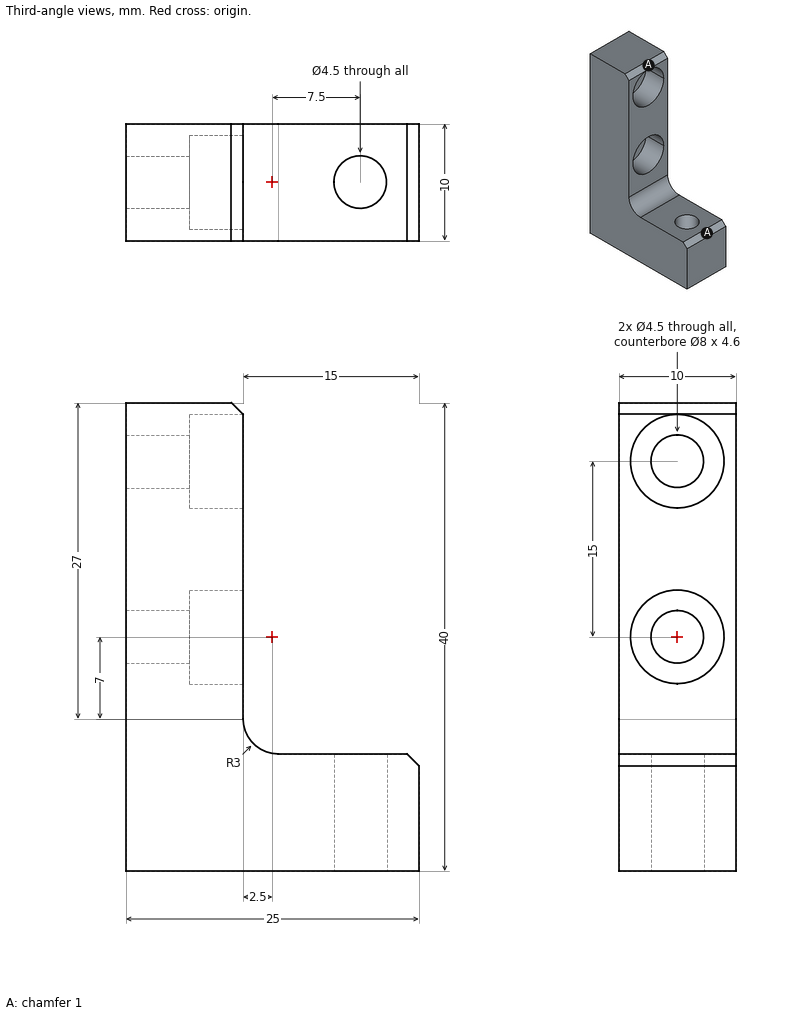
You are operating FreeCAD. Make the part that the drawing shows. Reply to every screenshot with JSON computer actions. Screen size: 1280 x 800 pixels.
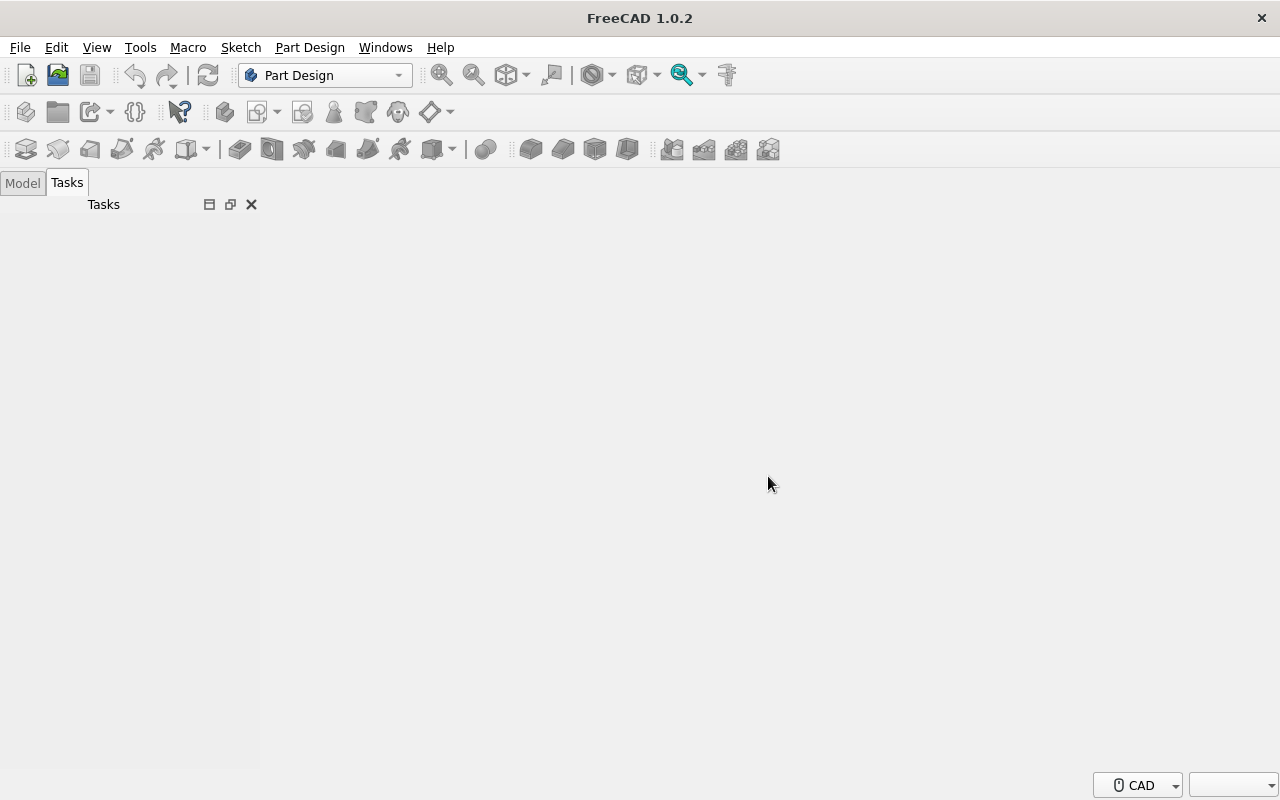
{"action": "left_click", "coordinate": [26, 76]}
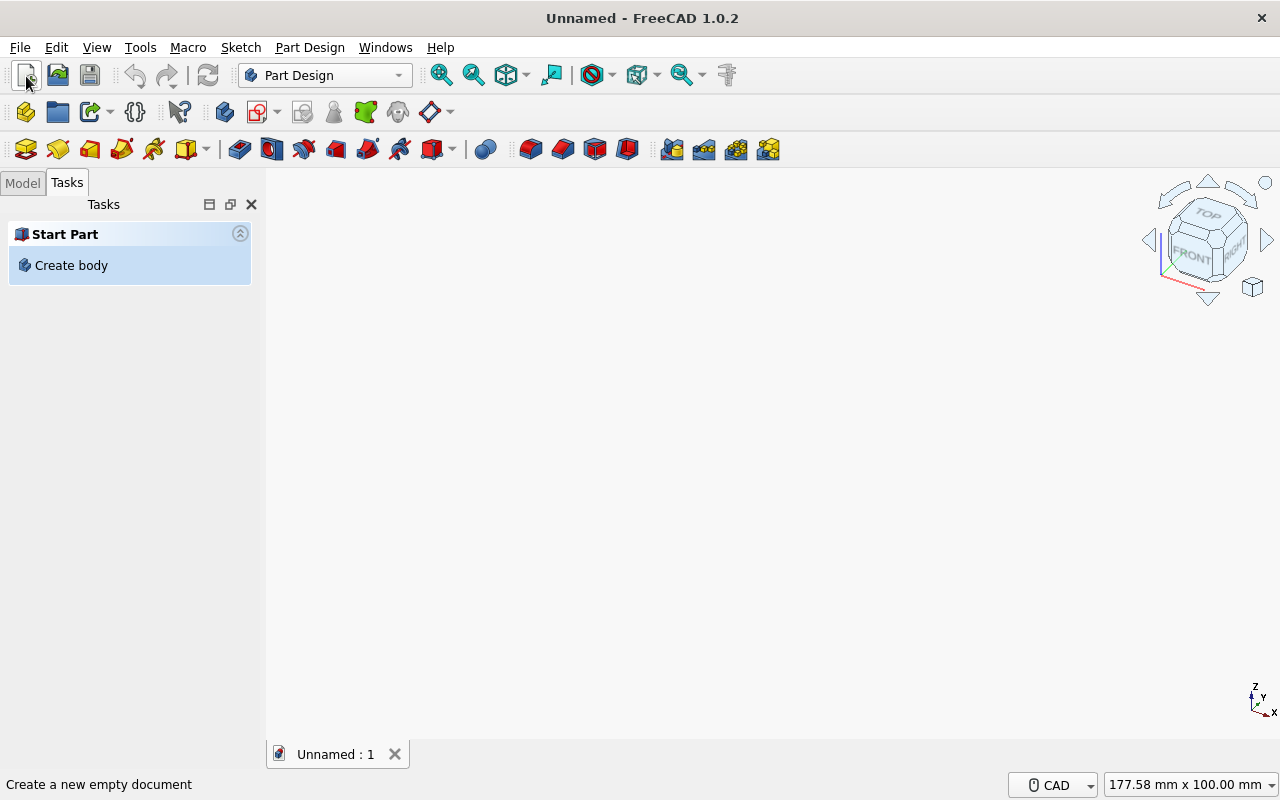
{"action": "left_click", "coordinate": [258, 112]}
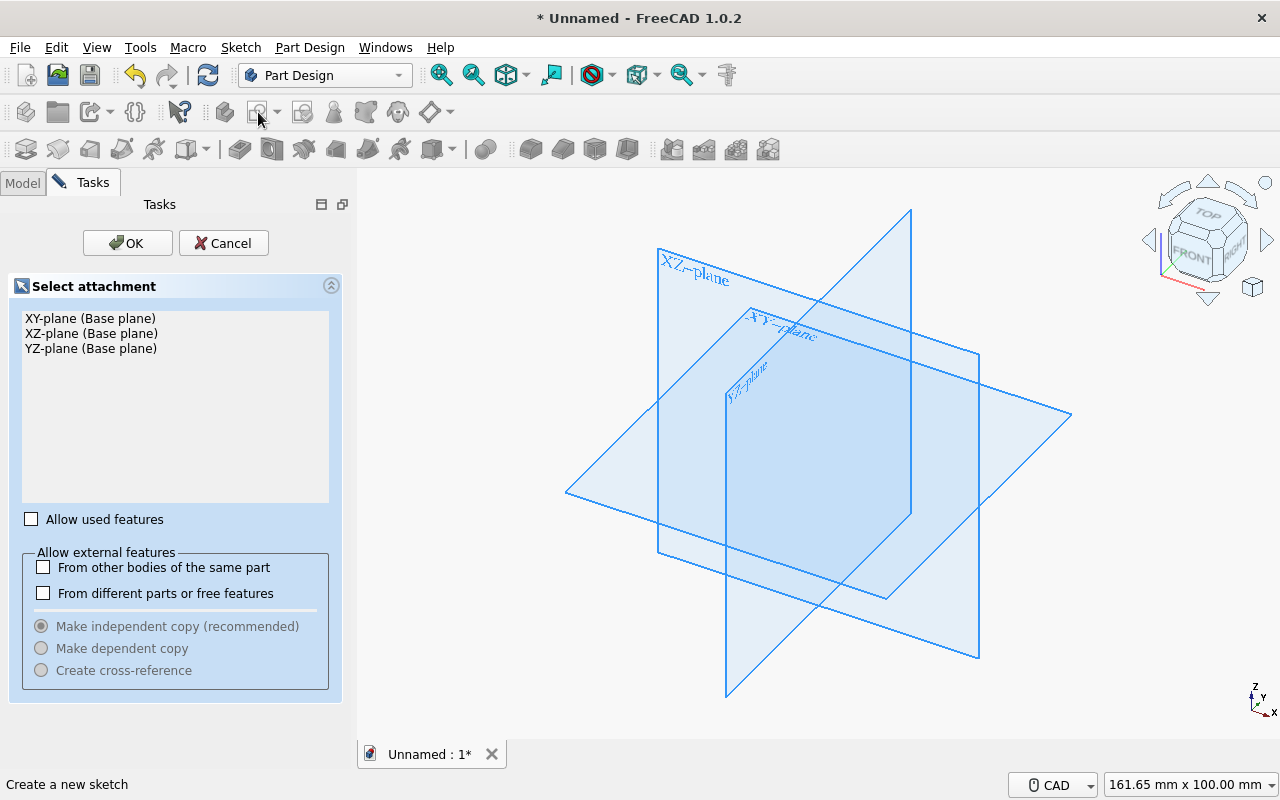
{"action": "left_click", "coordinate": [82, 334]}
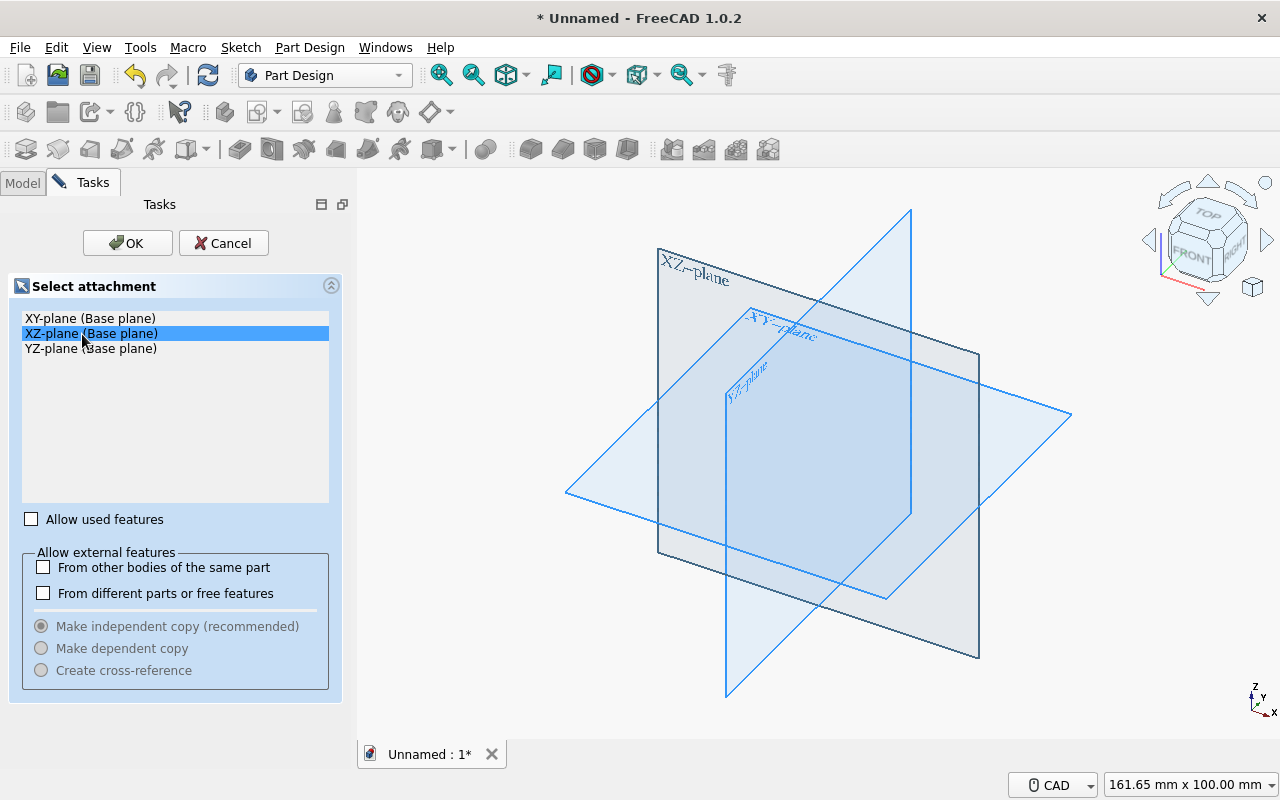
{"action": "left_click", "coordinate": [128, 243]}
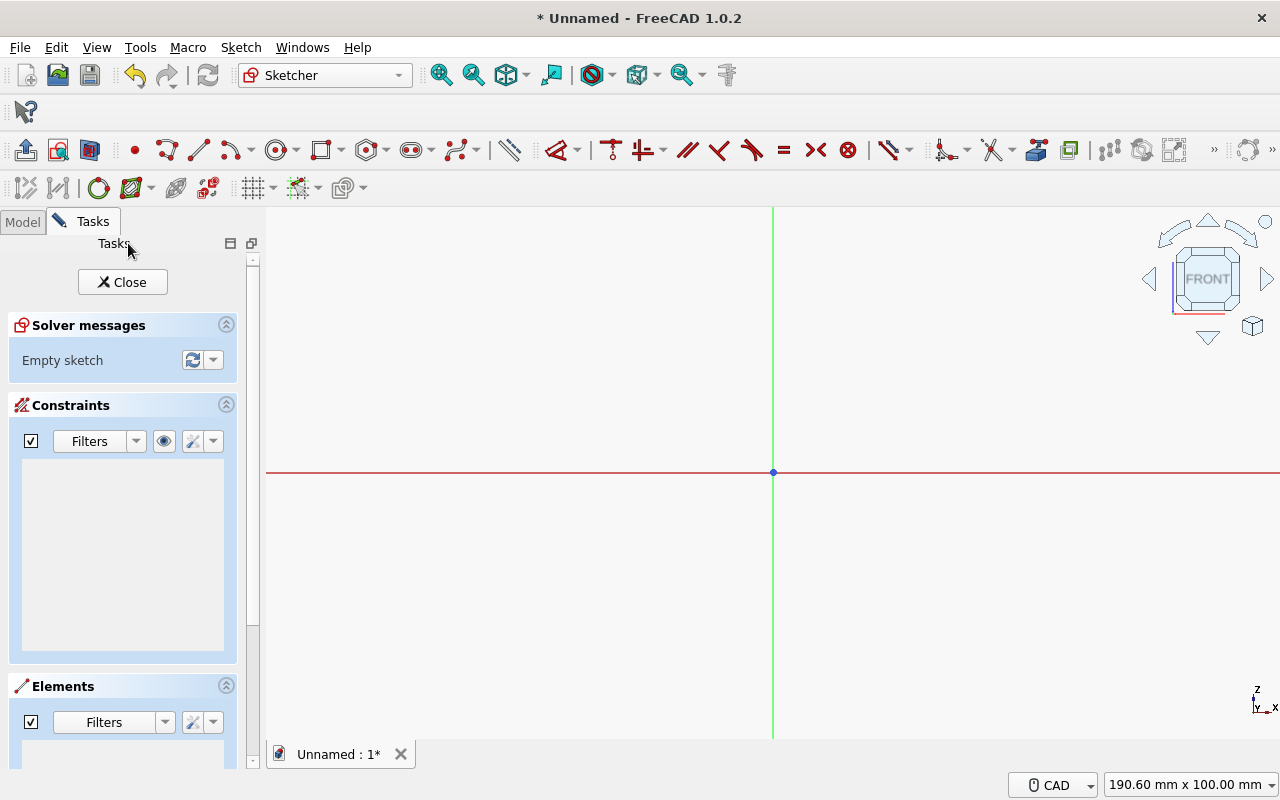
{"action": "scroll", "coordinate": [912, 473], "scroll_direction": "up", "scroll_amount": 2}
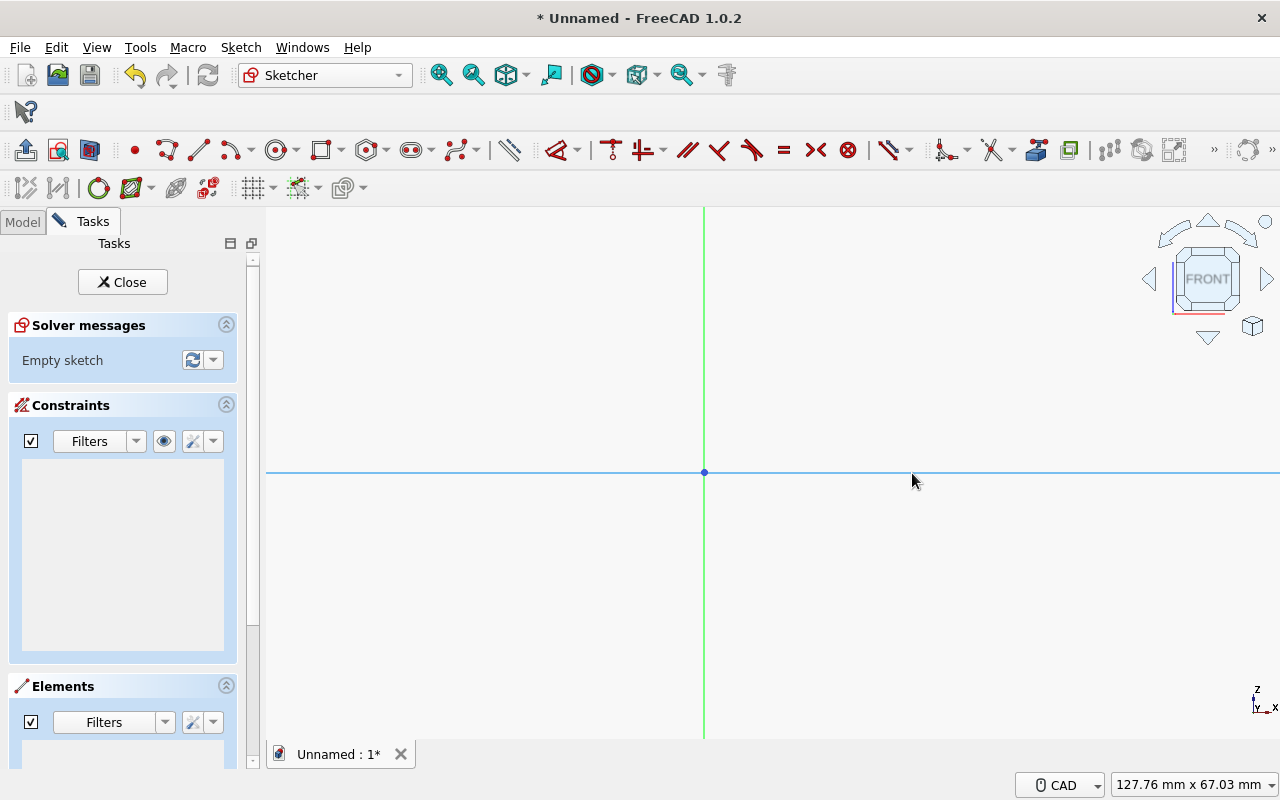
{"action": "left_click", "coordinate": [344, 150]}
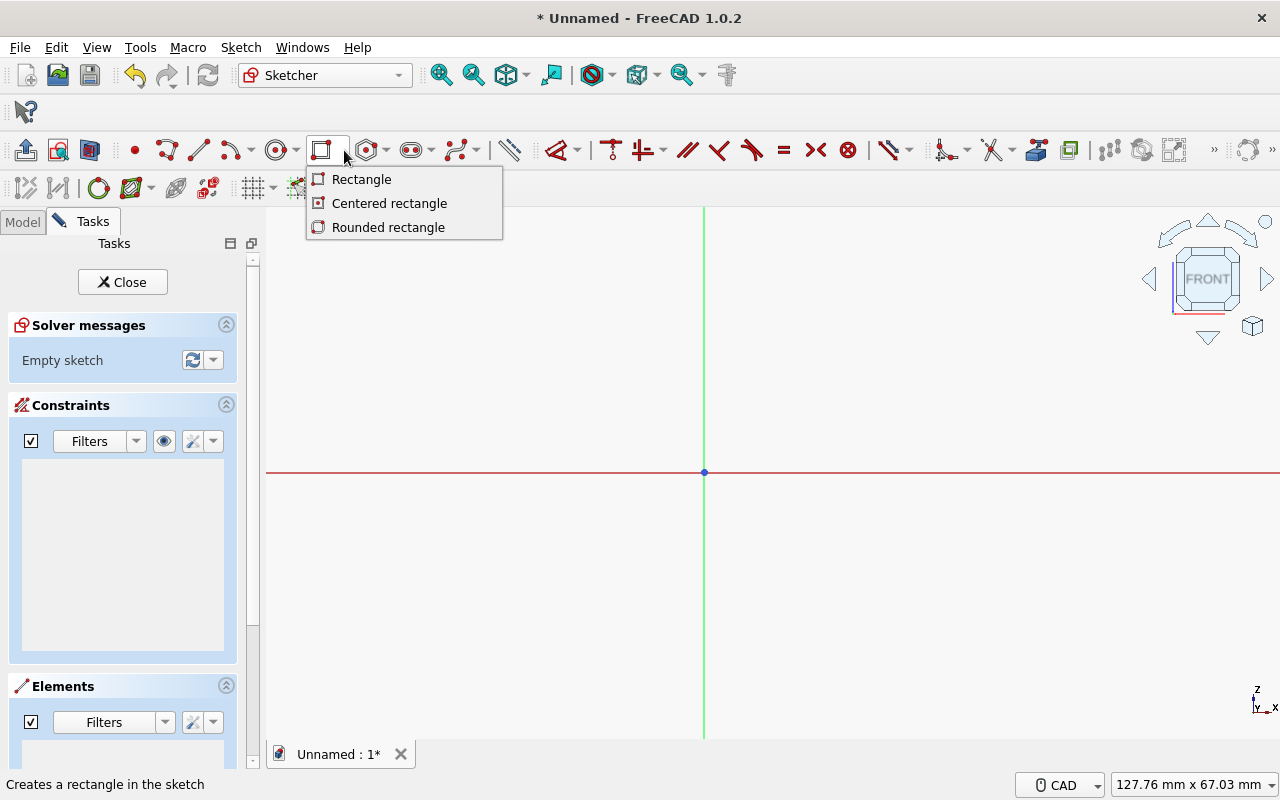
{"action": "left_click", "coordinate": [404, 203]}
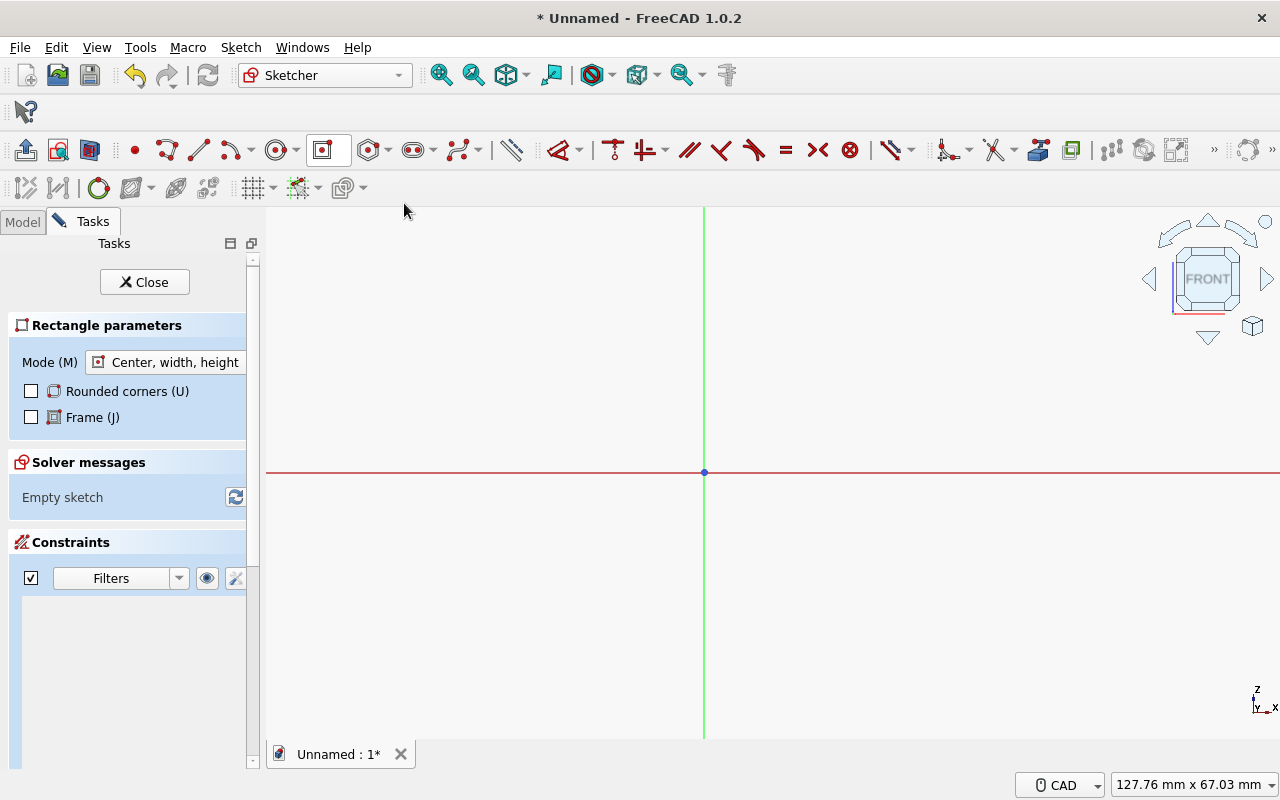
{"action": "left_click", "coordinate": [704, 473]}
{"action": "mouse_move", "coordinate": [804, 314]}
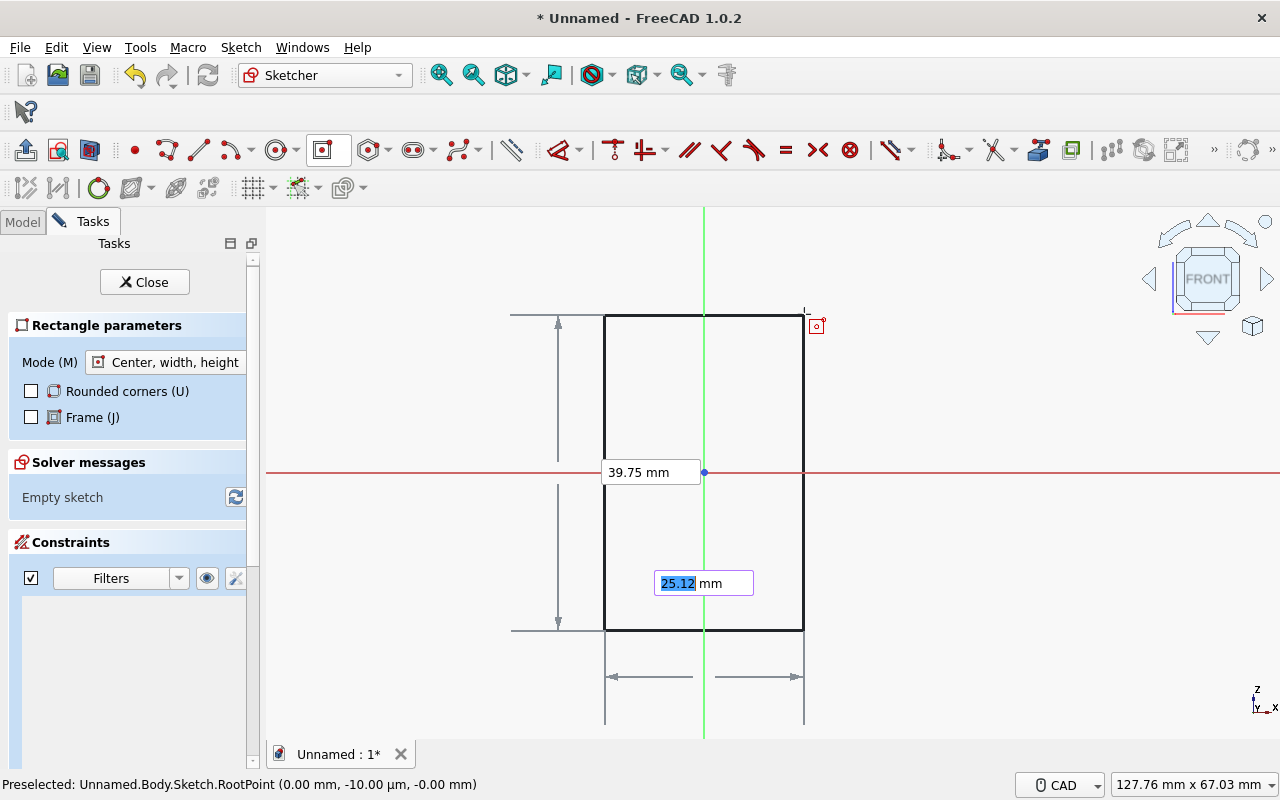
{"action": "type", "text": "25"}
{"action": "key", "text": "Tab"}
{"action": "type", "text": "40"}
{"action": "key", "text": "Return"}
{"action": "key", "text": "Escape"}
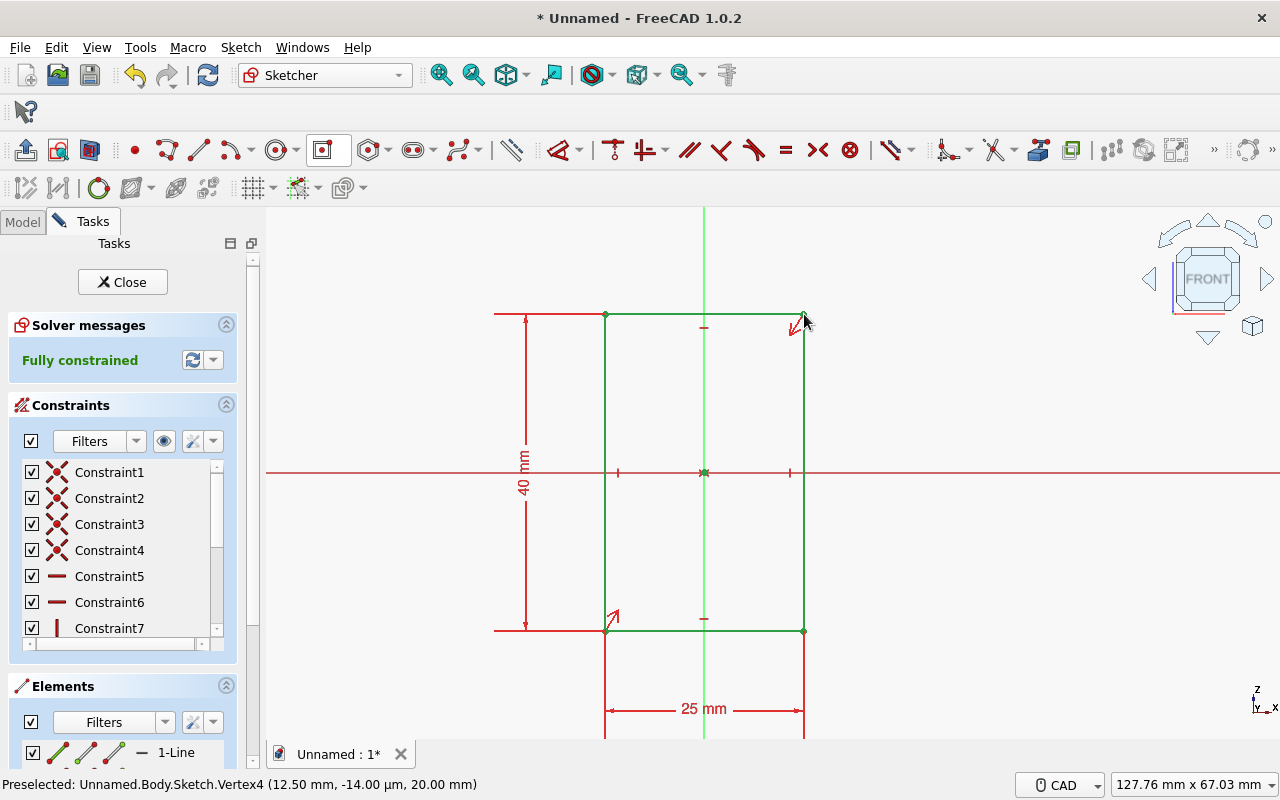
{"action": "left_click", "coordinate": [123, 282]}